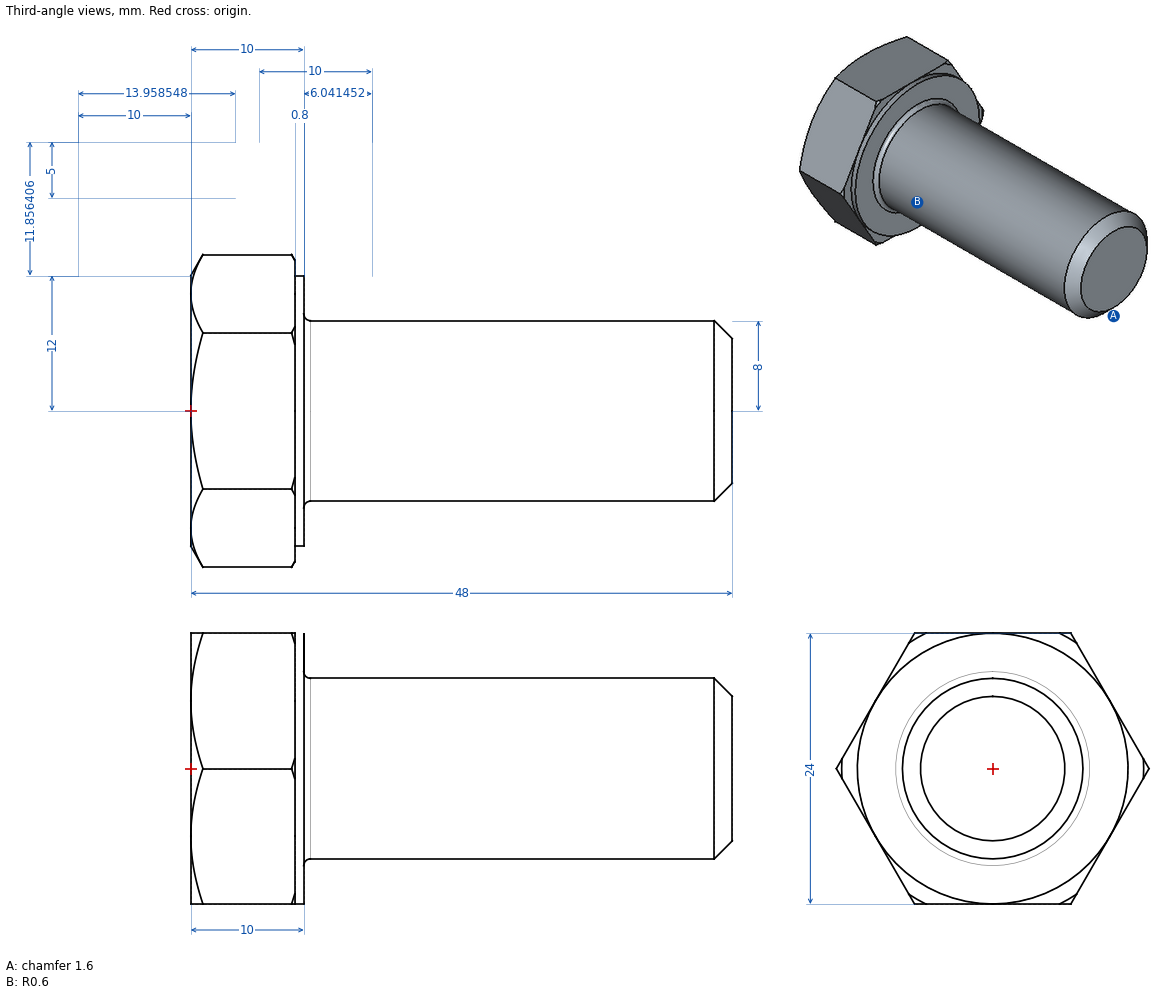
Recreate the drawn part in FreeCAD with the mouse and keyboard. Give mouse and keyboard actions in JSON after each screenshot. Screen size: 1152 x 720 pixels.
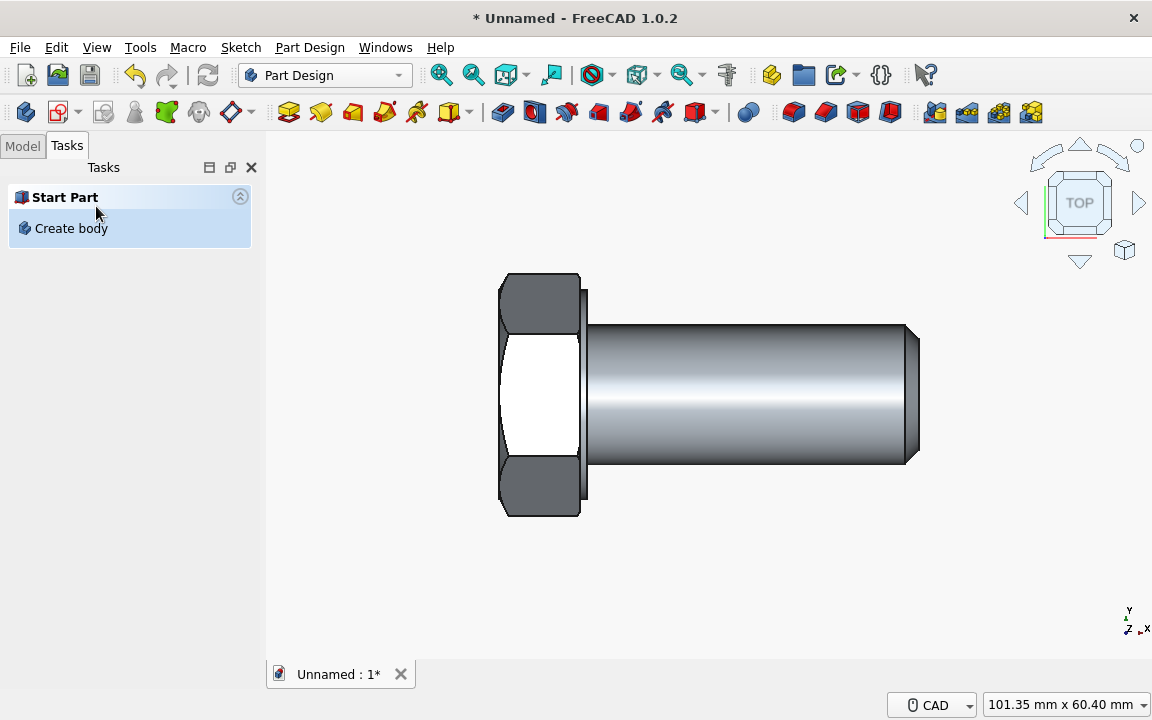
{"action": "key", "text": "1"}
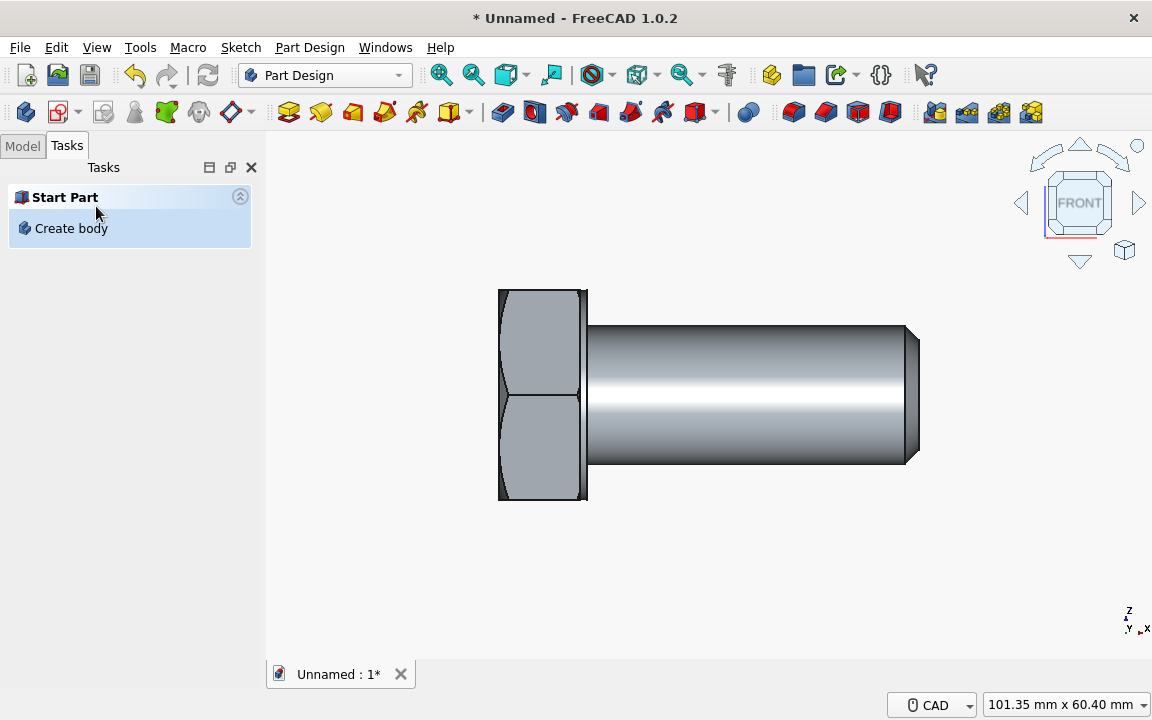
{"action": "key", "text": "3"}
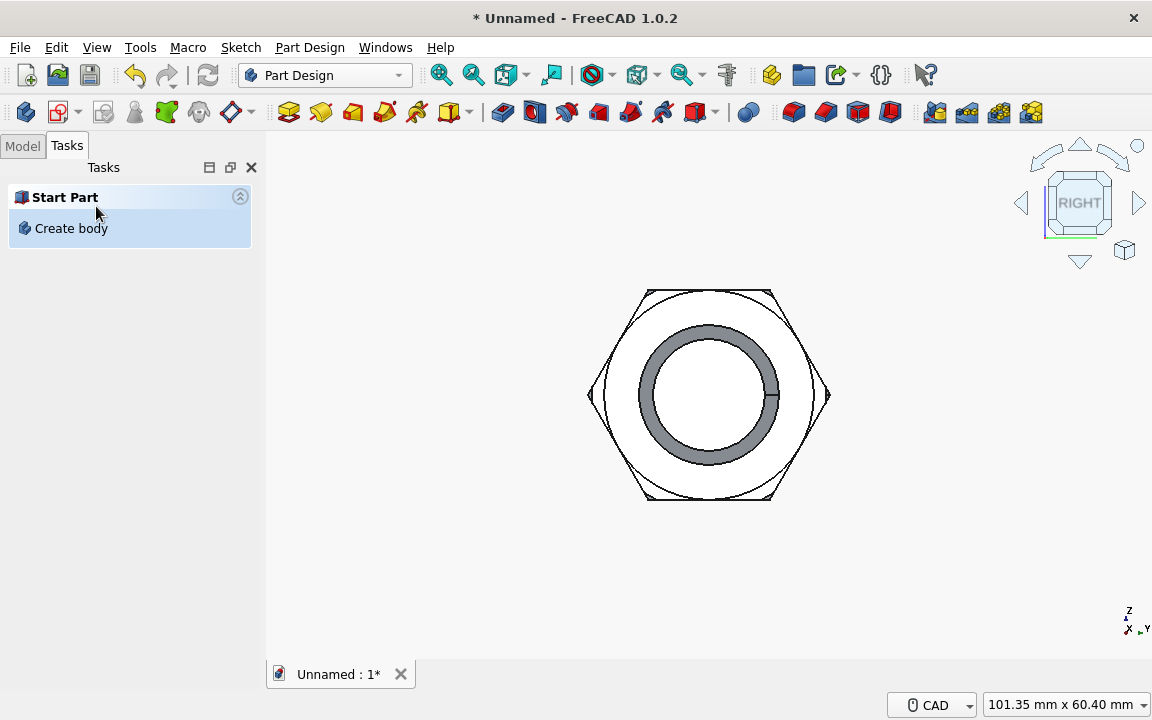
{"action": "left_click", "coordinate": [442, 76]}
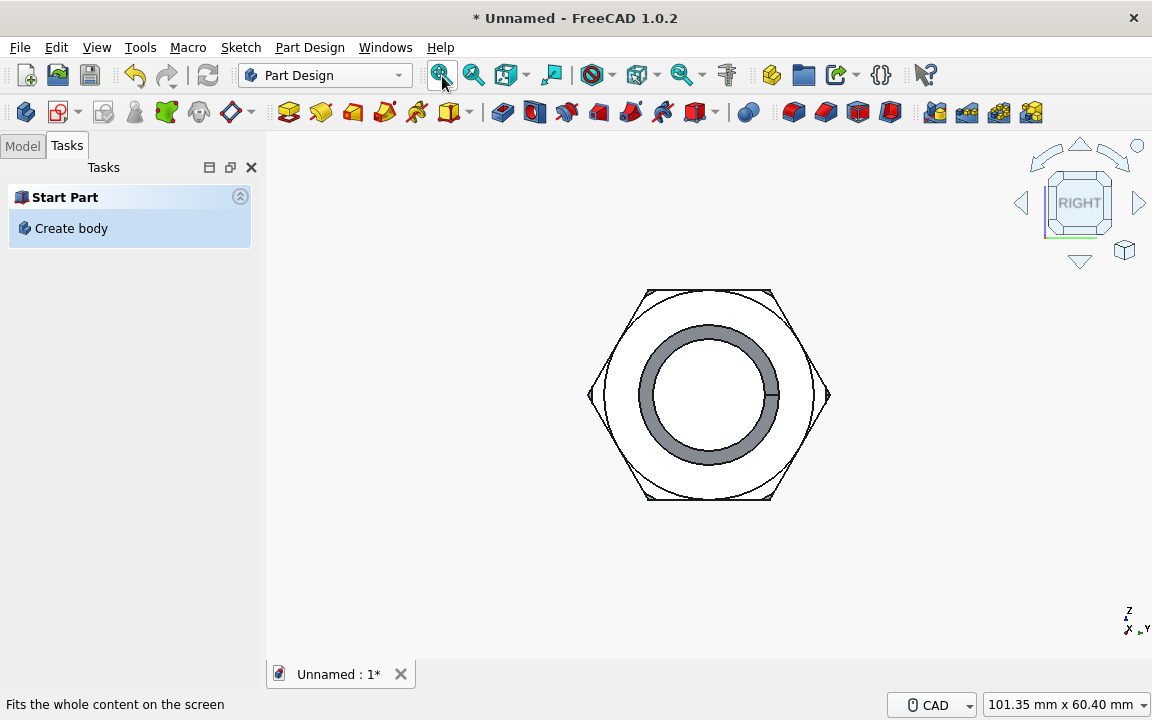
{"action": "key", "text": "5"}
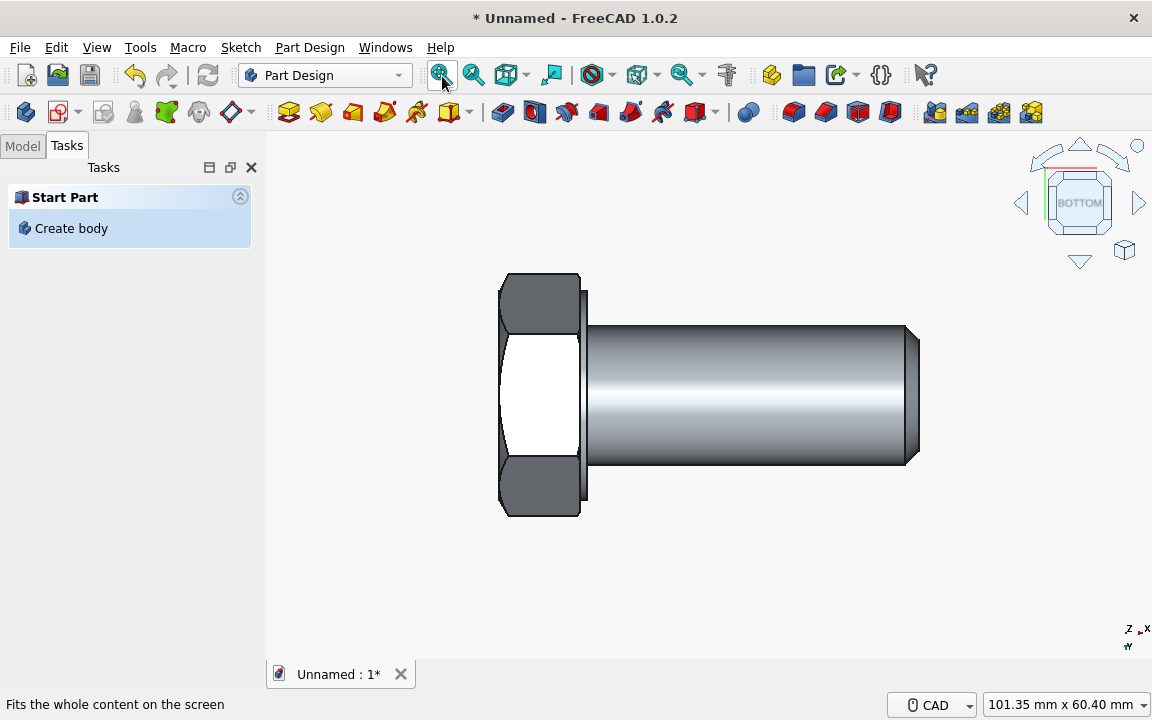
{"action": "key", "text": "4"}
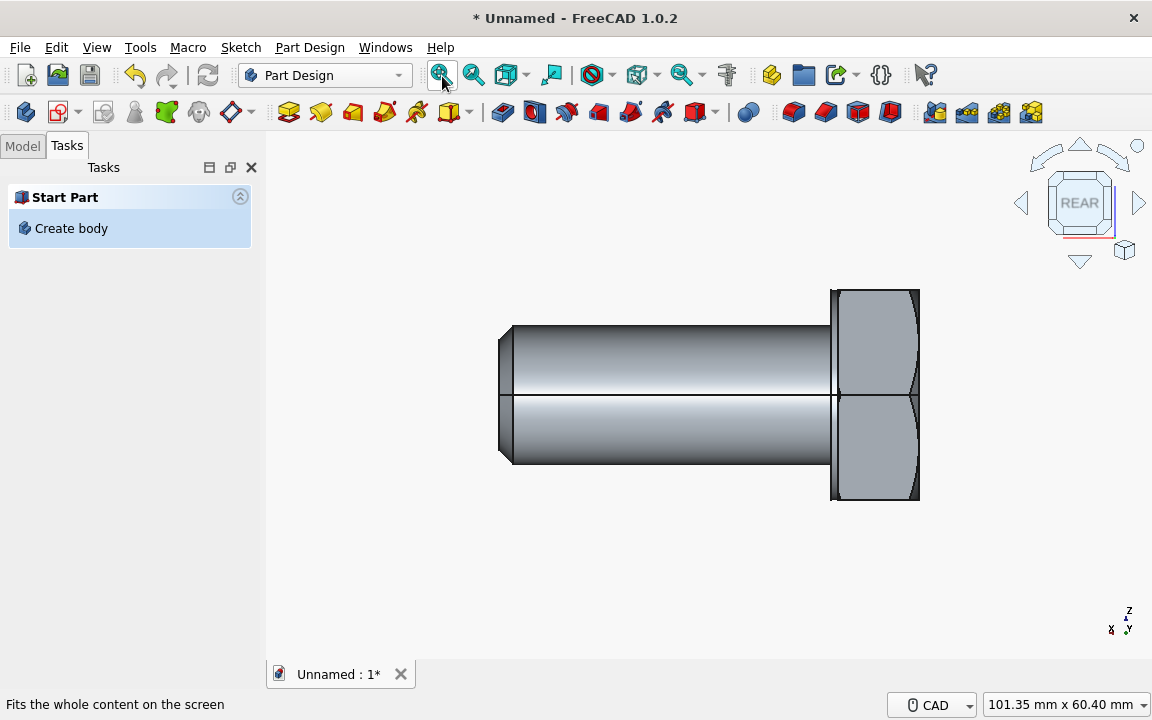
{"action": "key", "text": "6"}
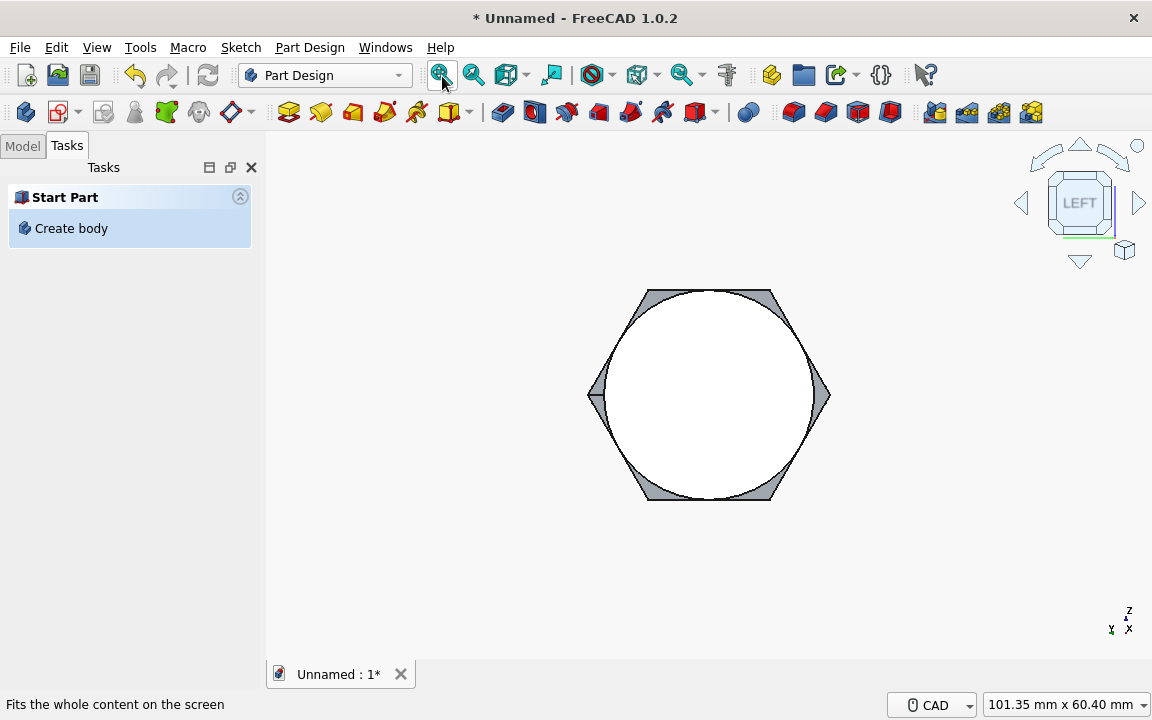
{"action": "left_click", "coordinate": [442, 76]}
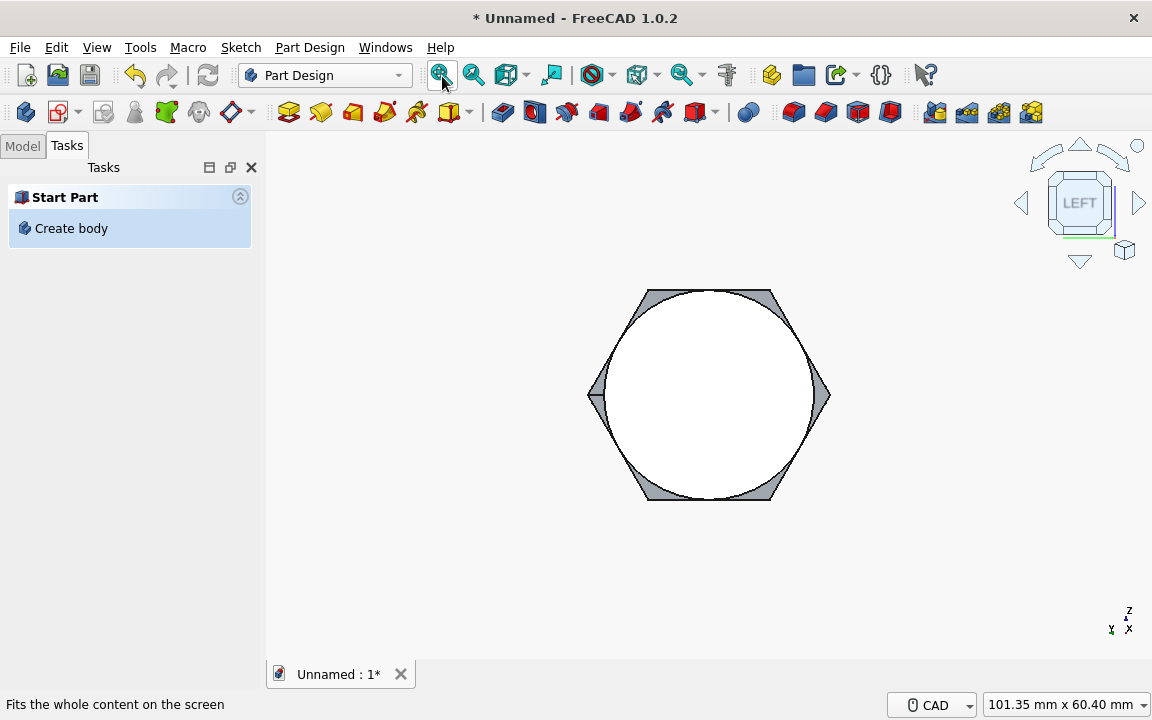
{"action": "key", "text": "v 3"}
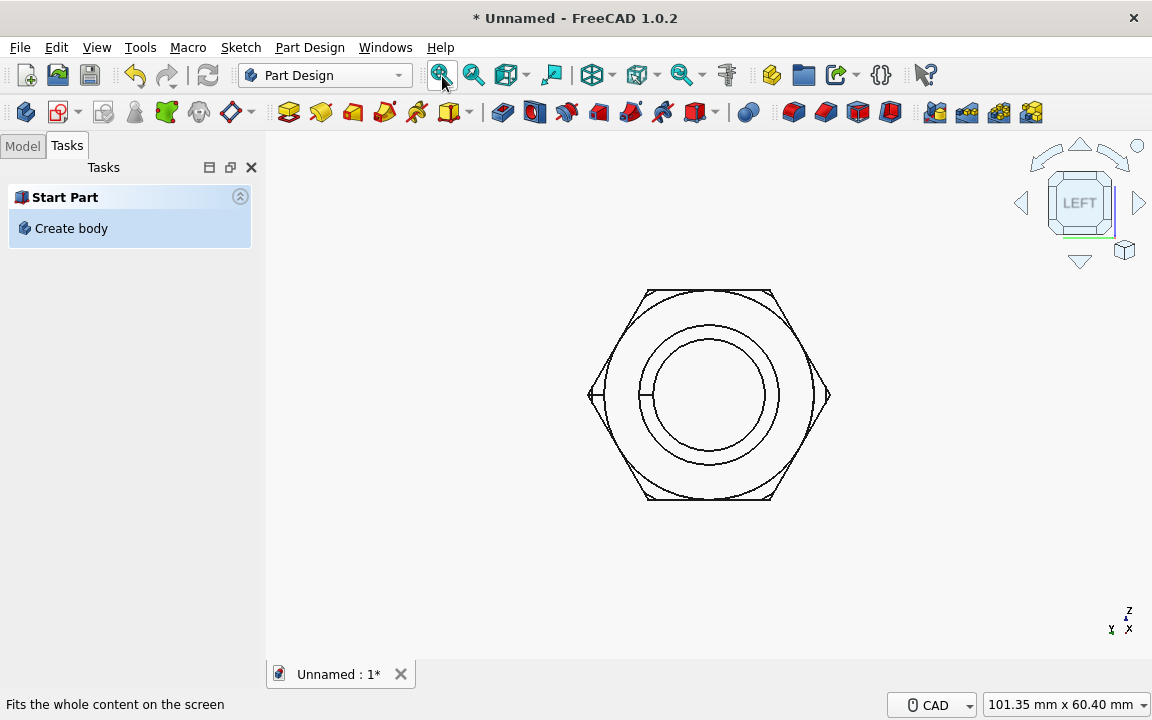
{"action": "key", "text": "0"}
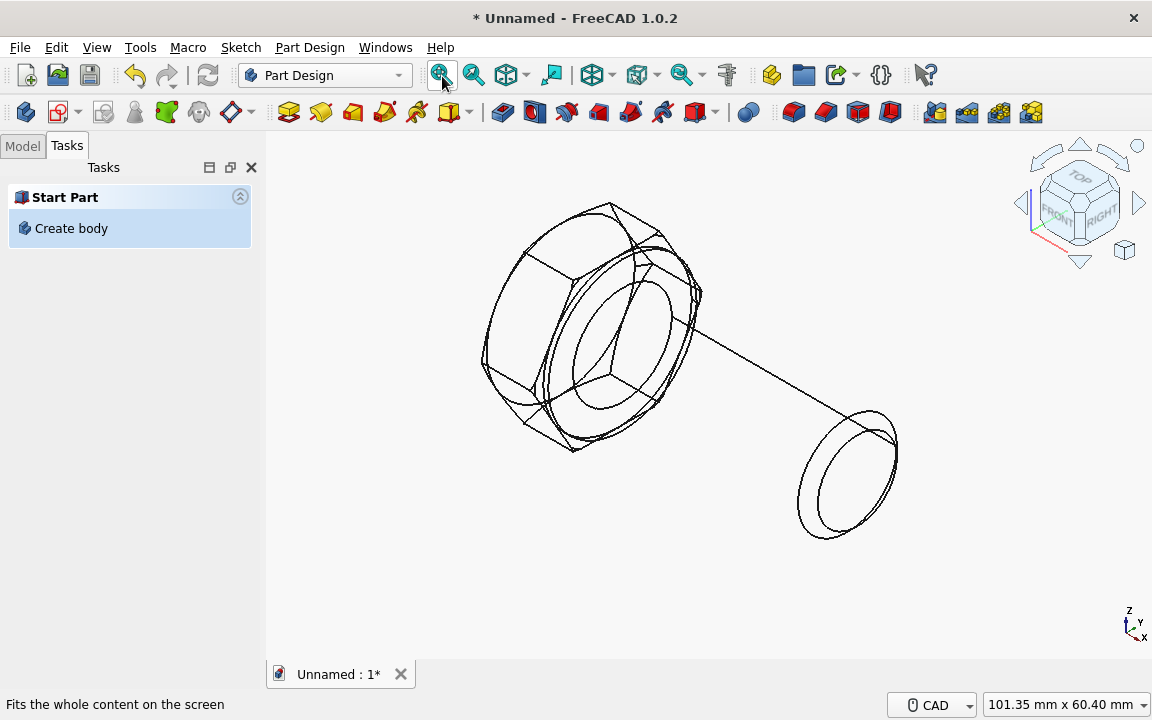
{"action": "left_click", "coordinate": [573, 373]}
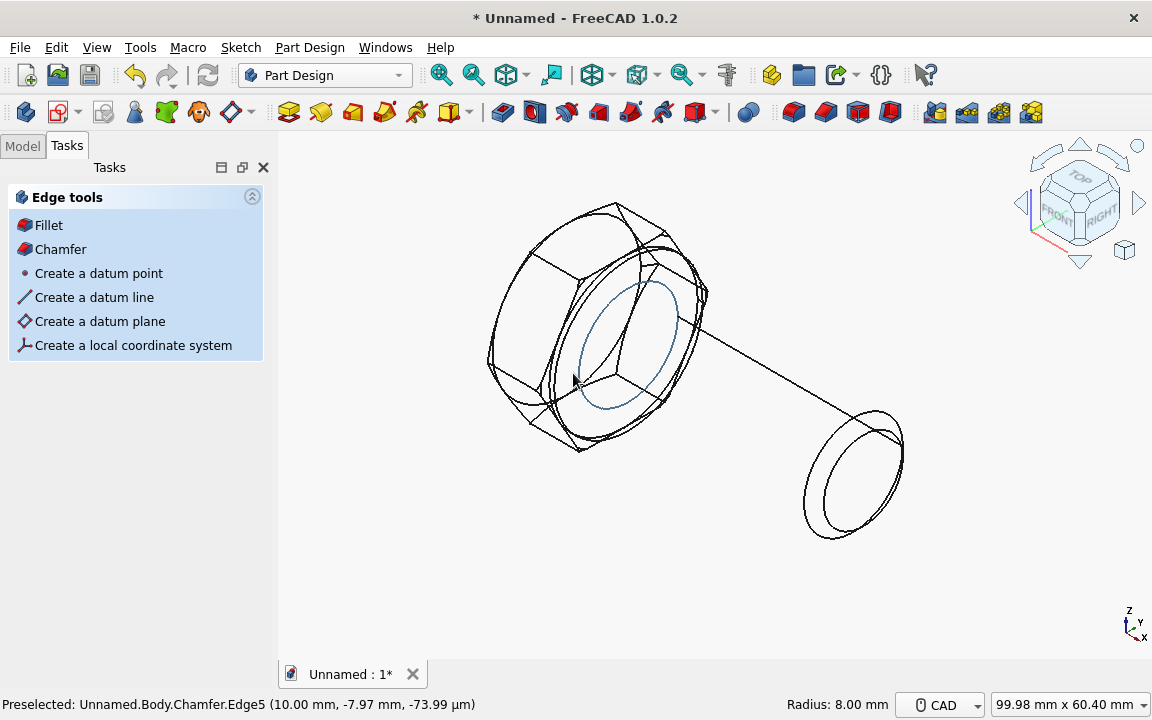
{"action": "key", "text": "v 1"}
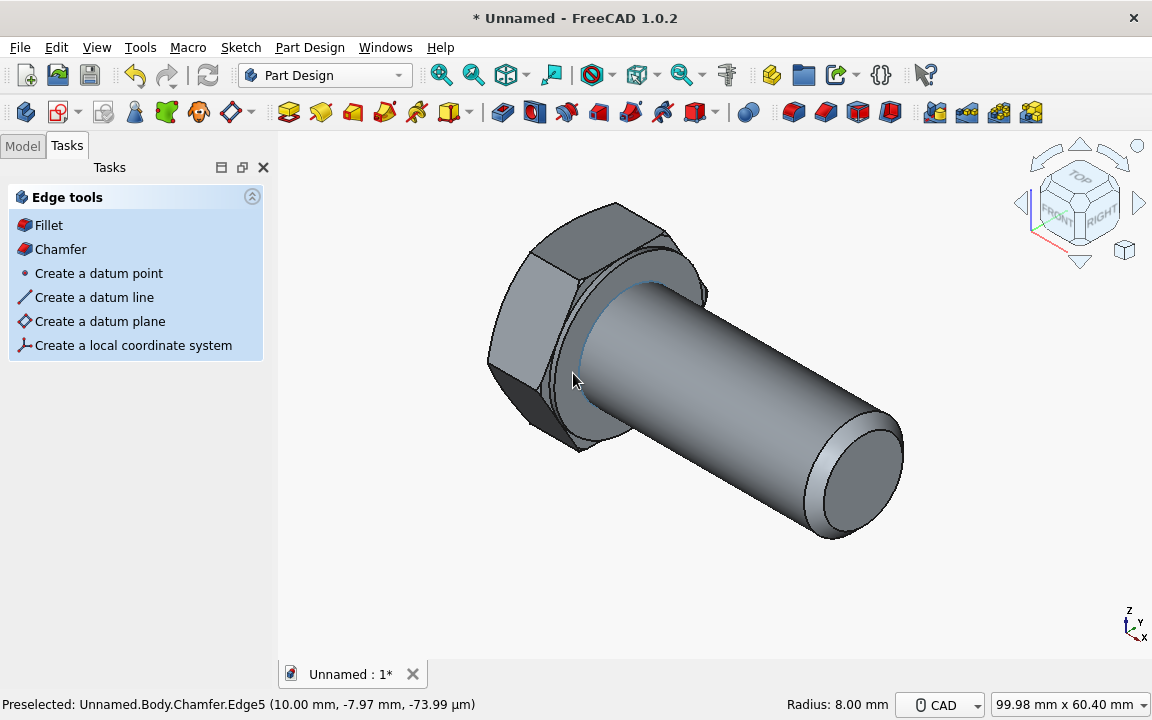
{"action": "left_click", "coordinate": [794, 112]}